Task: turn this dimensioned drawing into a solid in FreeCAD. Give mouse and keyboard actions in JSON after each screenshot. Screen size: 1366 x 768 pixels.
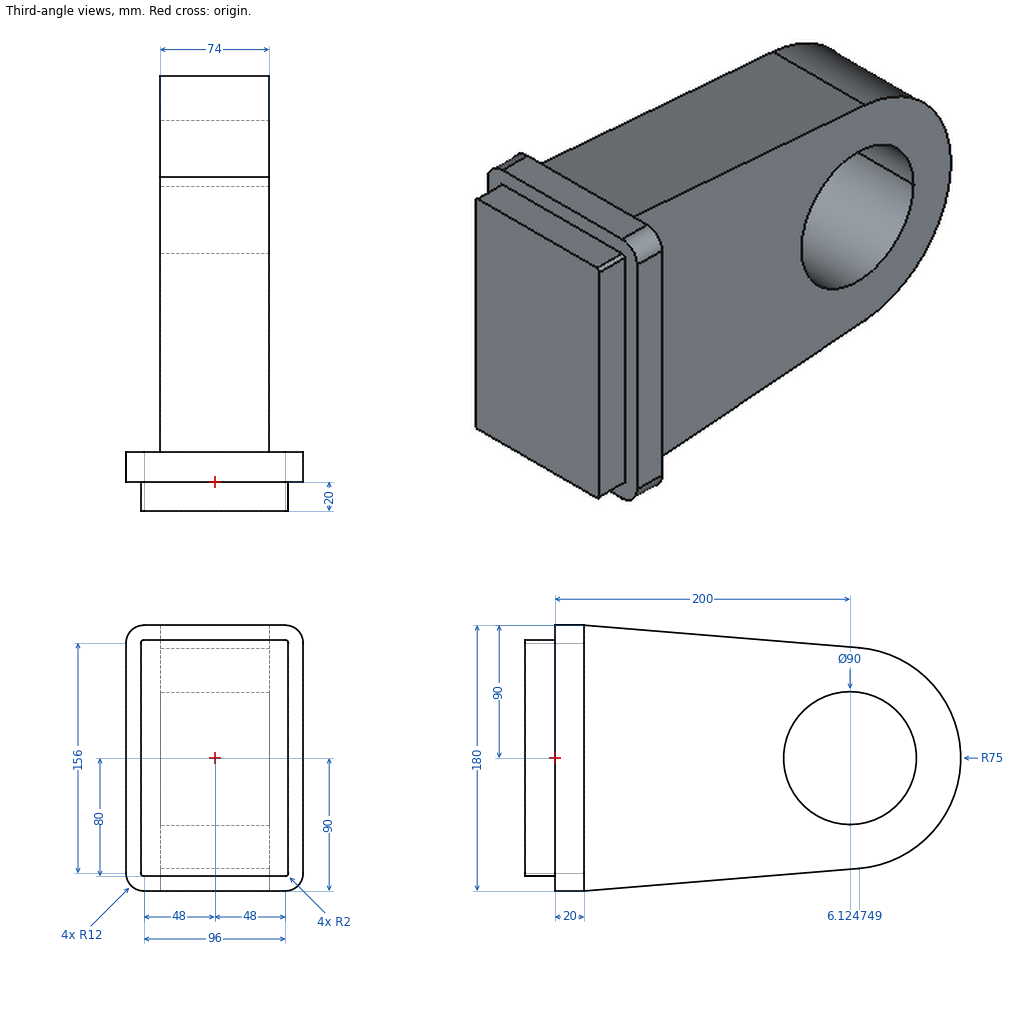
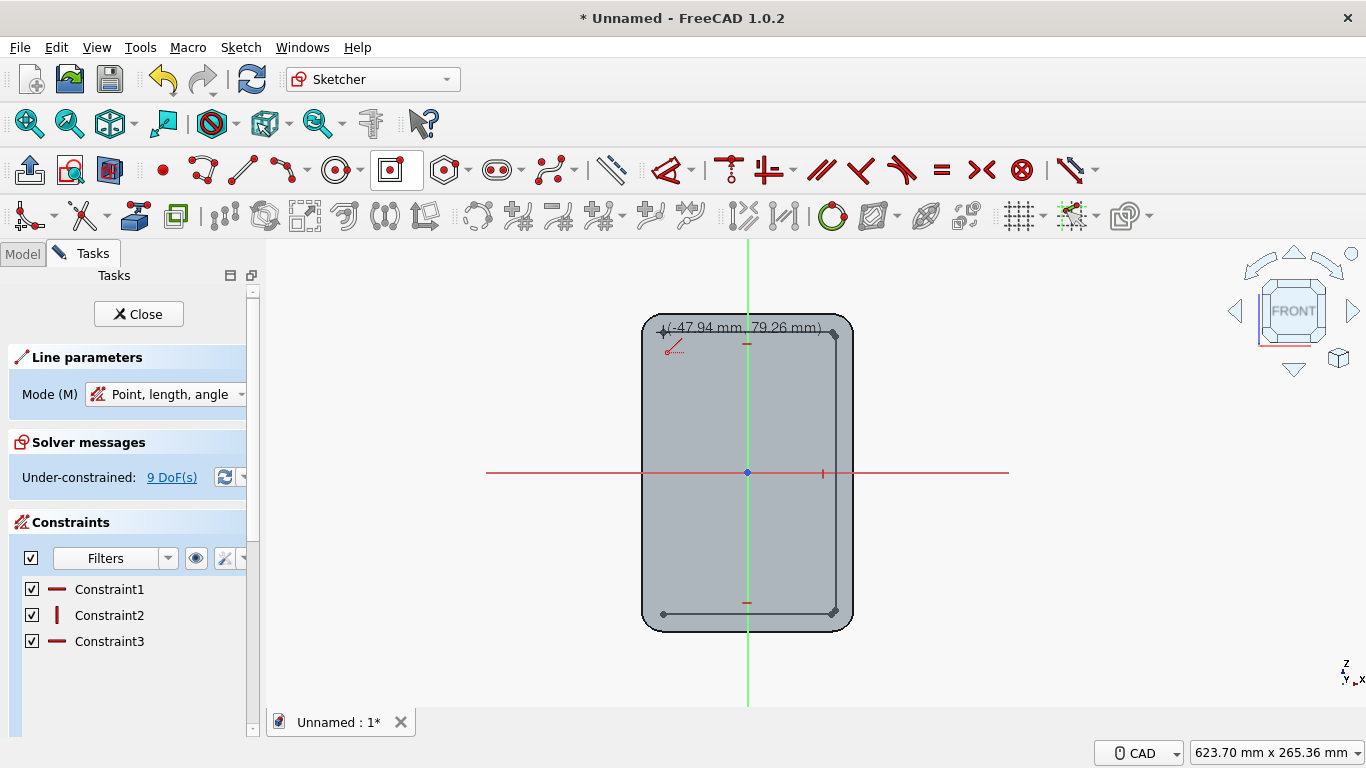
{"action": "scroll", "coordinate": [659, 335], "scroll_direction": "up", "scroll_amount": 6}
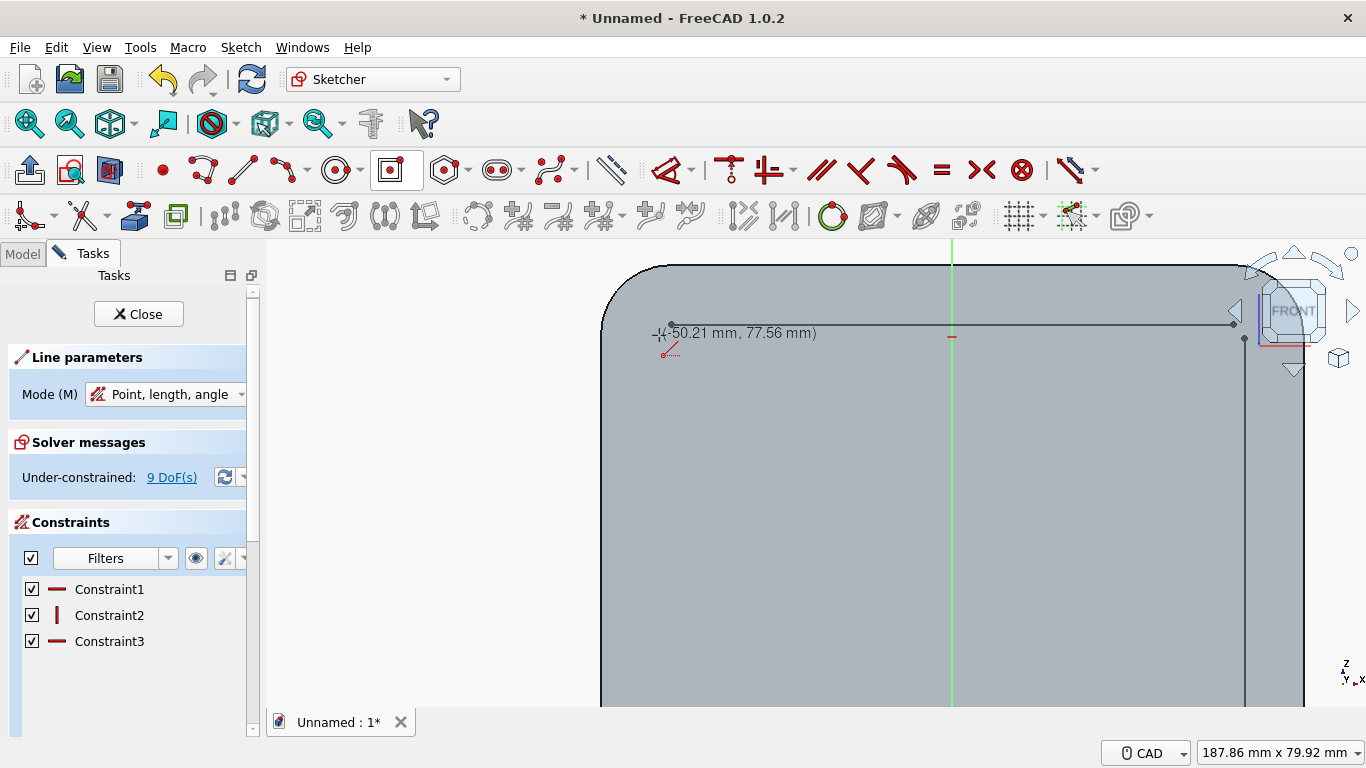
{"action": "left_click", "coordinate": [659, 335]}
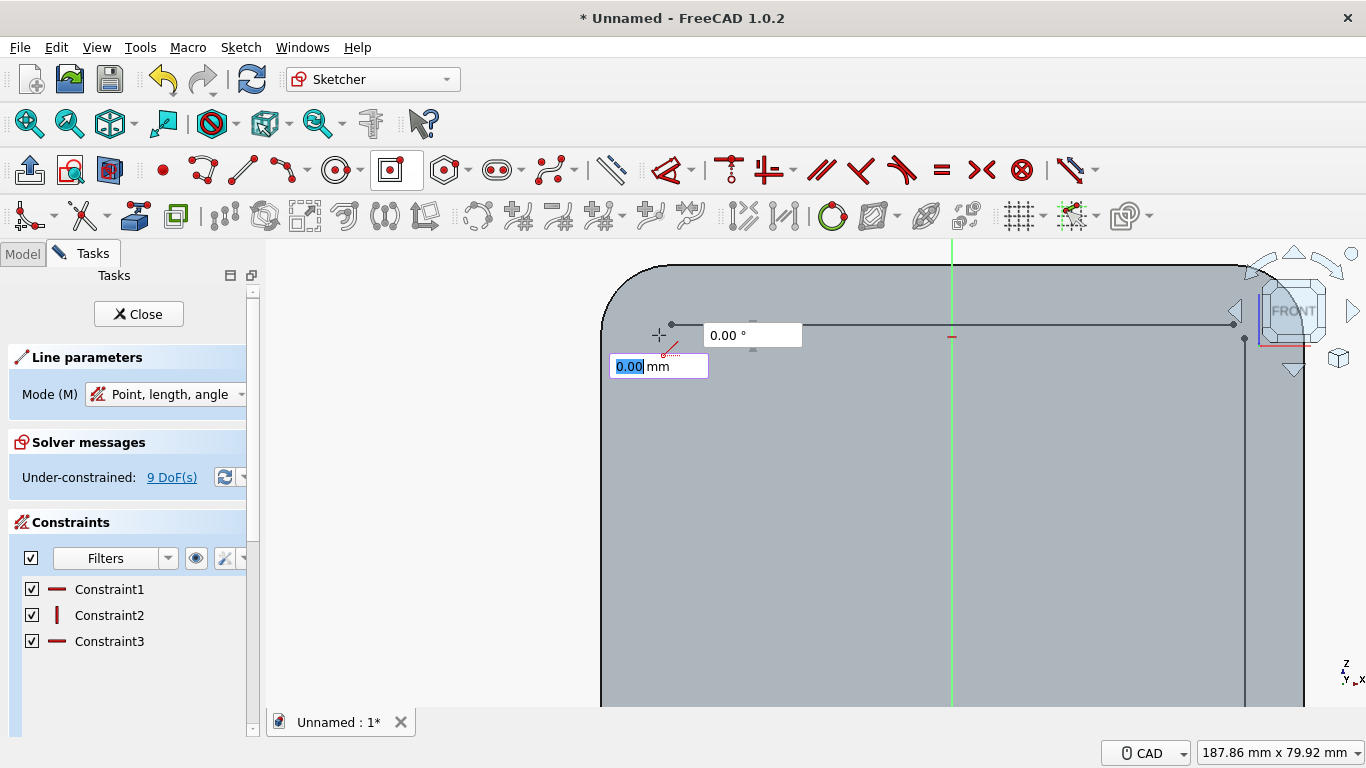
{"action": "scroll", "coordinate": [659, 335], "scroll_direction": "down", "scroll_amount": 6}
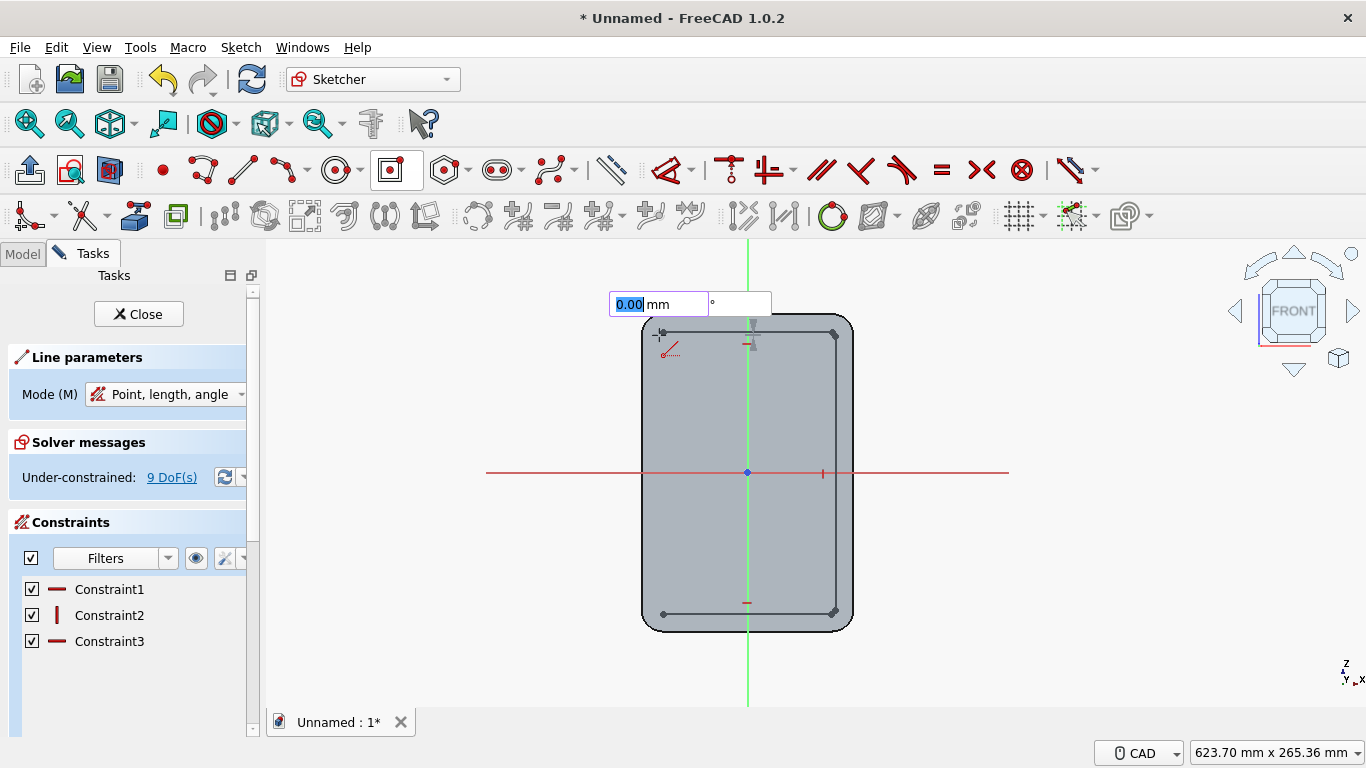
{"action": "scroll", "coordinate": [659, 610], "scroll_direction": "up", "scroll_amount": 6}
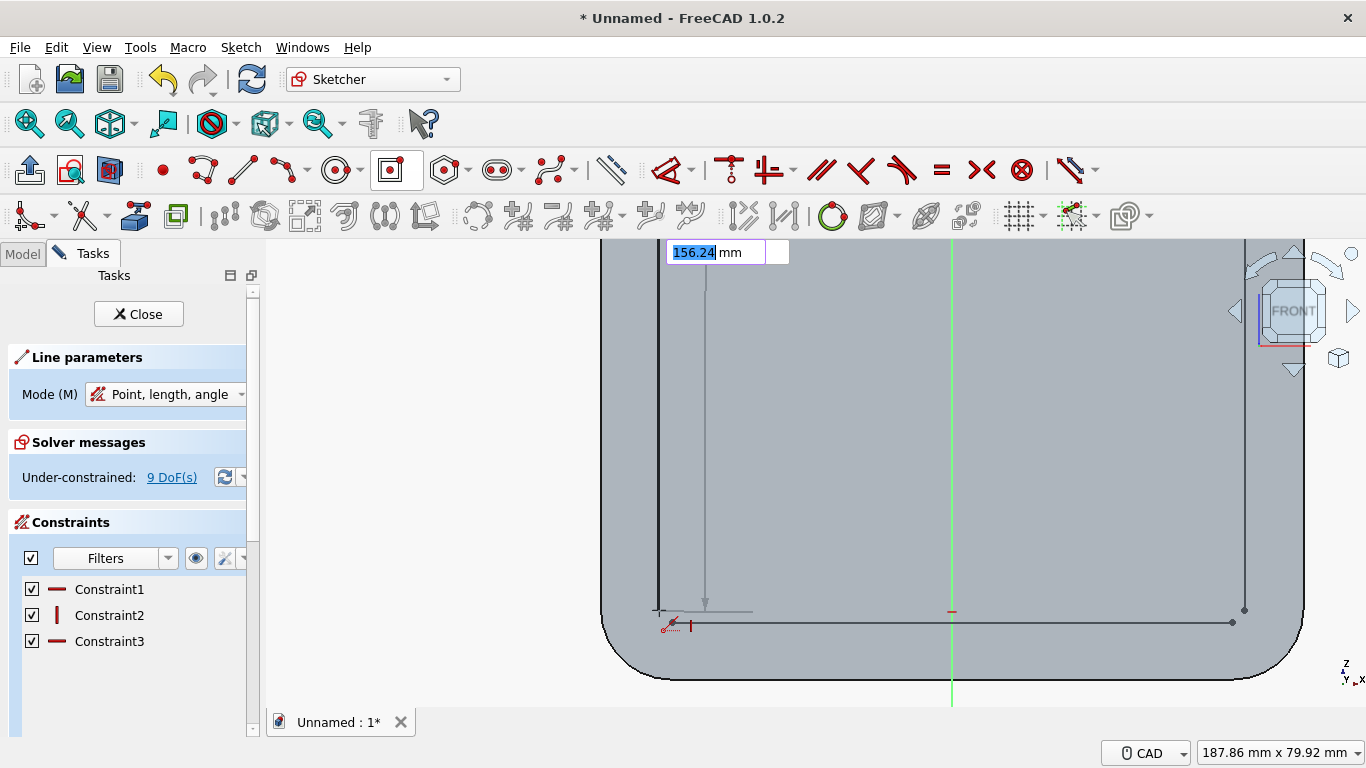
{"action": "left_click", "coordinate": [659, 609]}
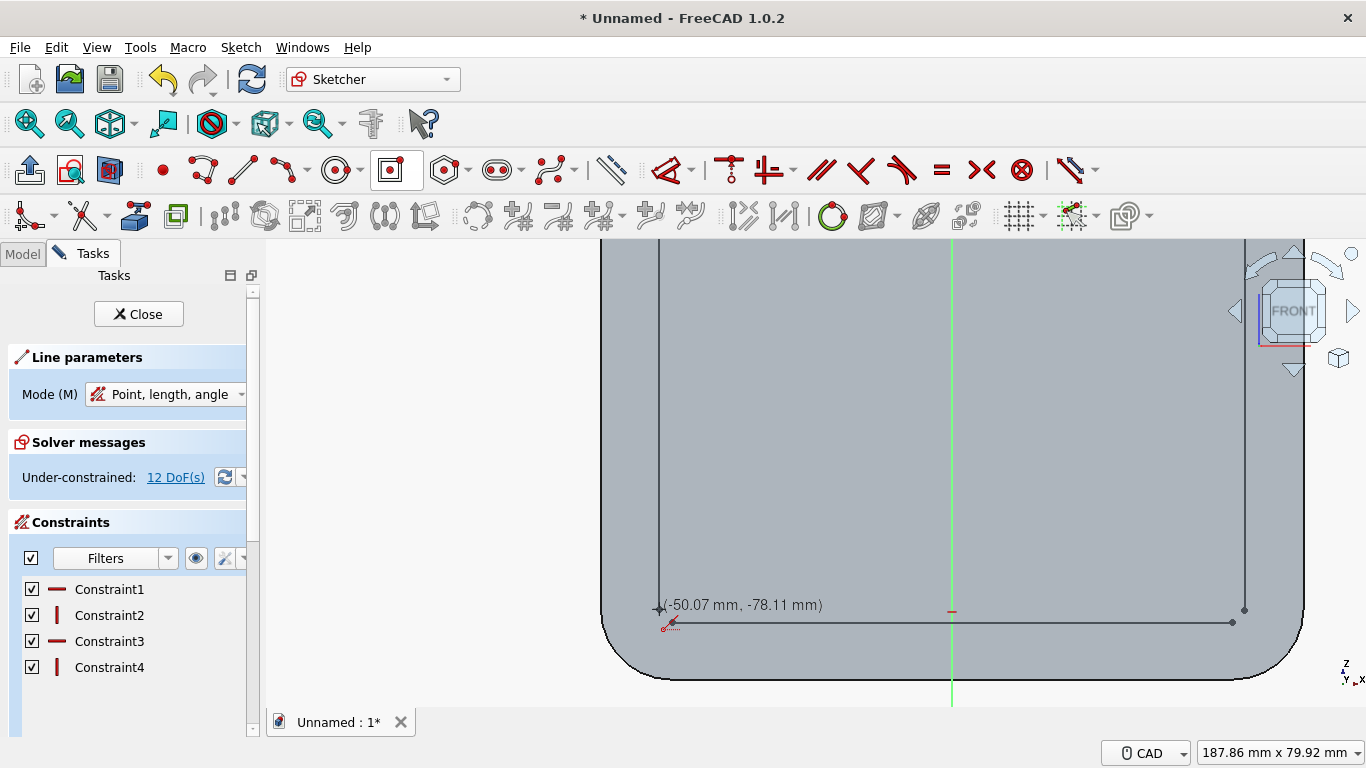
{"action": "left_click", "coordinate": [284, 170]}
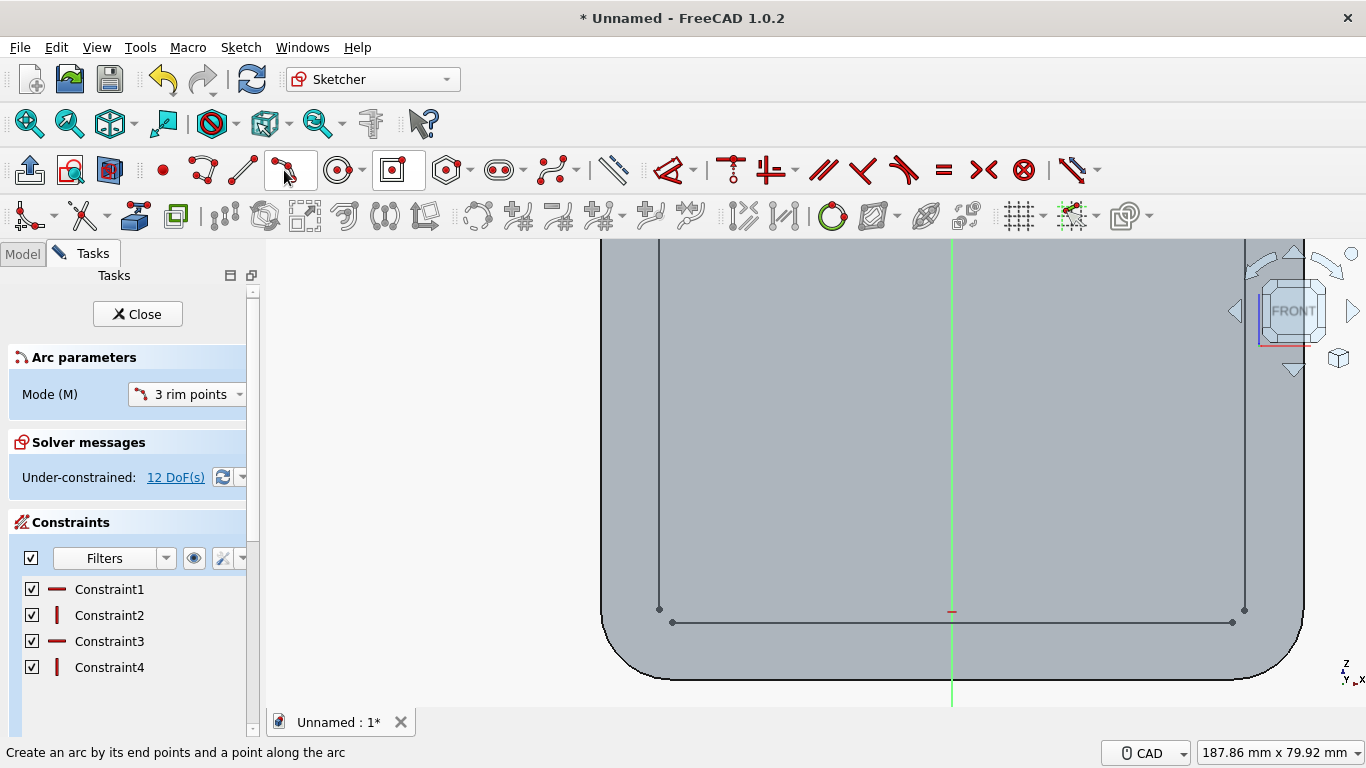
{"action": "scroll", "coordinate": [659, 611], "scroll_direction": "down", "scroll_amount": 6}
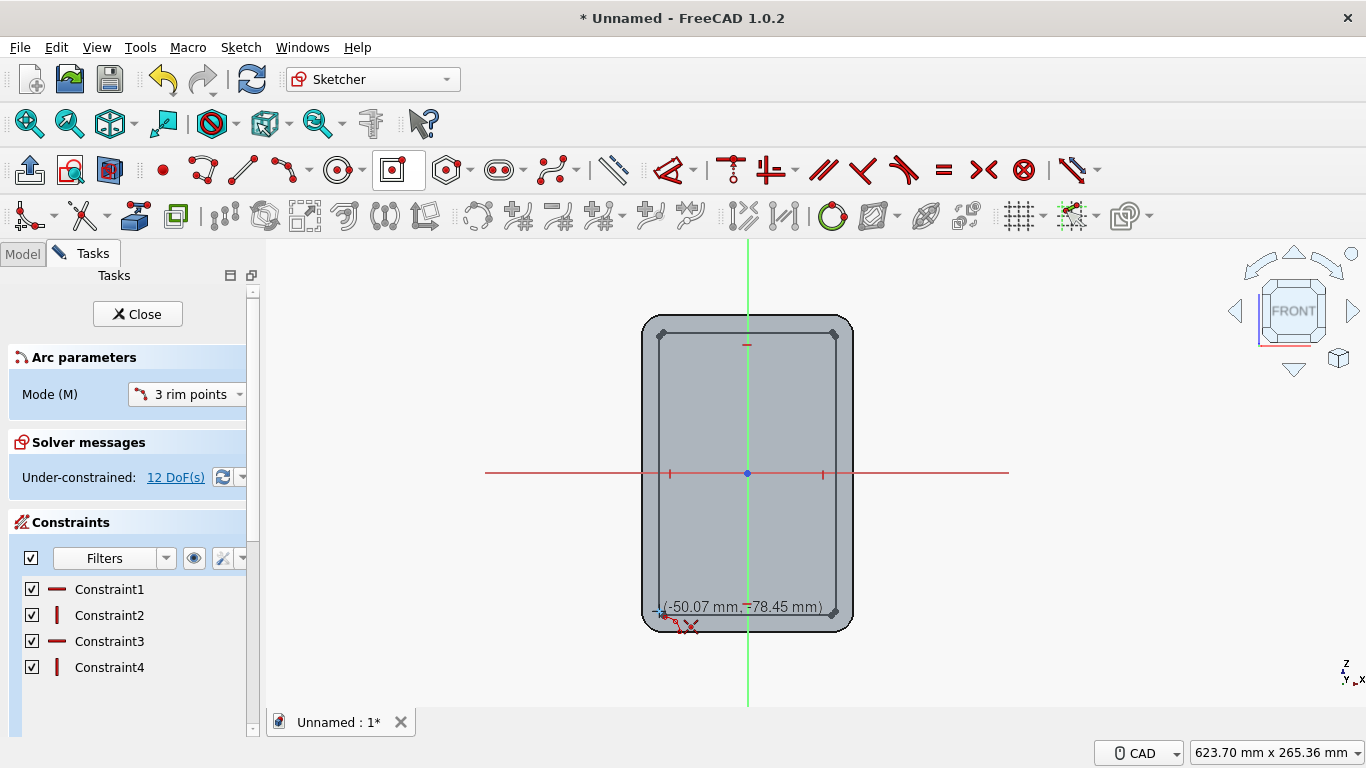
{"action": "scroll", "coordinate": [832, 615], "scroll_direction": "up", "scroll_amount": 6}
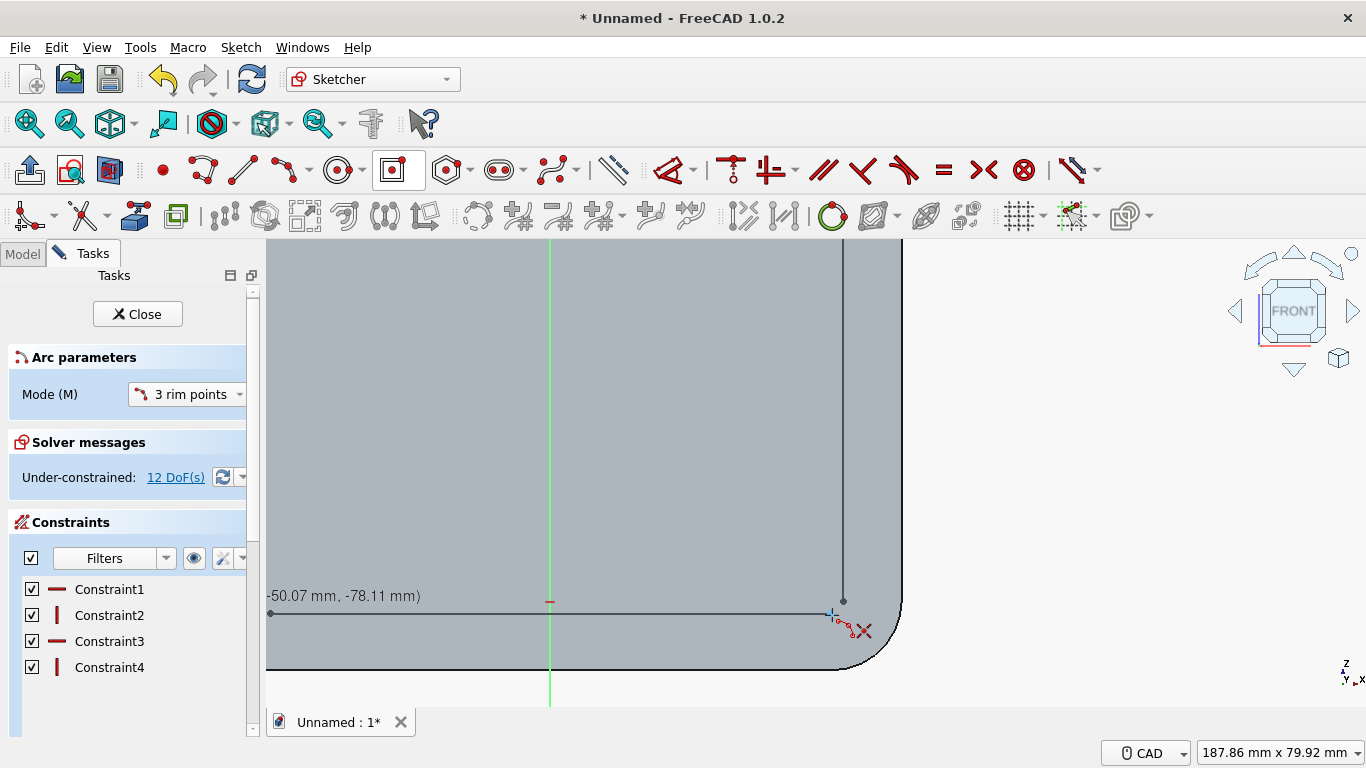
{"action": "left_click", "coordinate": [830, 614]}
{"action": "left_click", "coordinate": [843, 601]}